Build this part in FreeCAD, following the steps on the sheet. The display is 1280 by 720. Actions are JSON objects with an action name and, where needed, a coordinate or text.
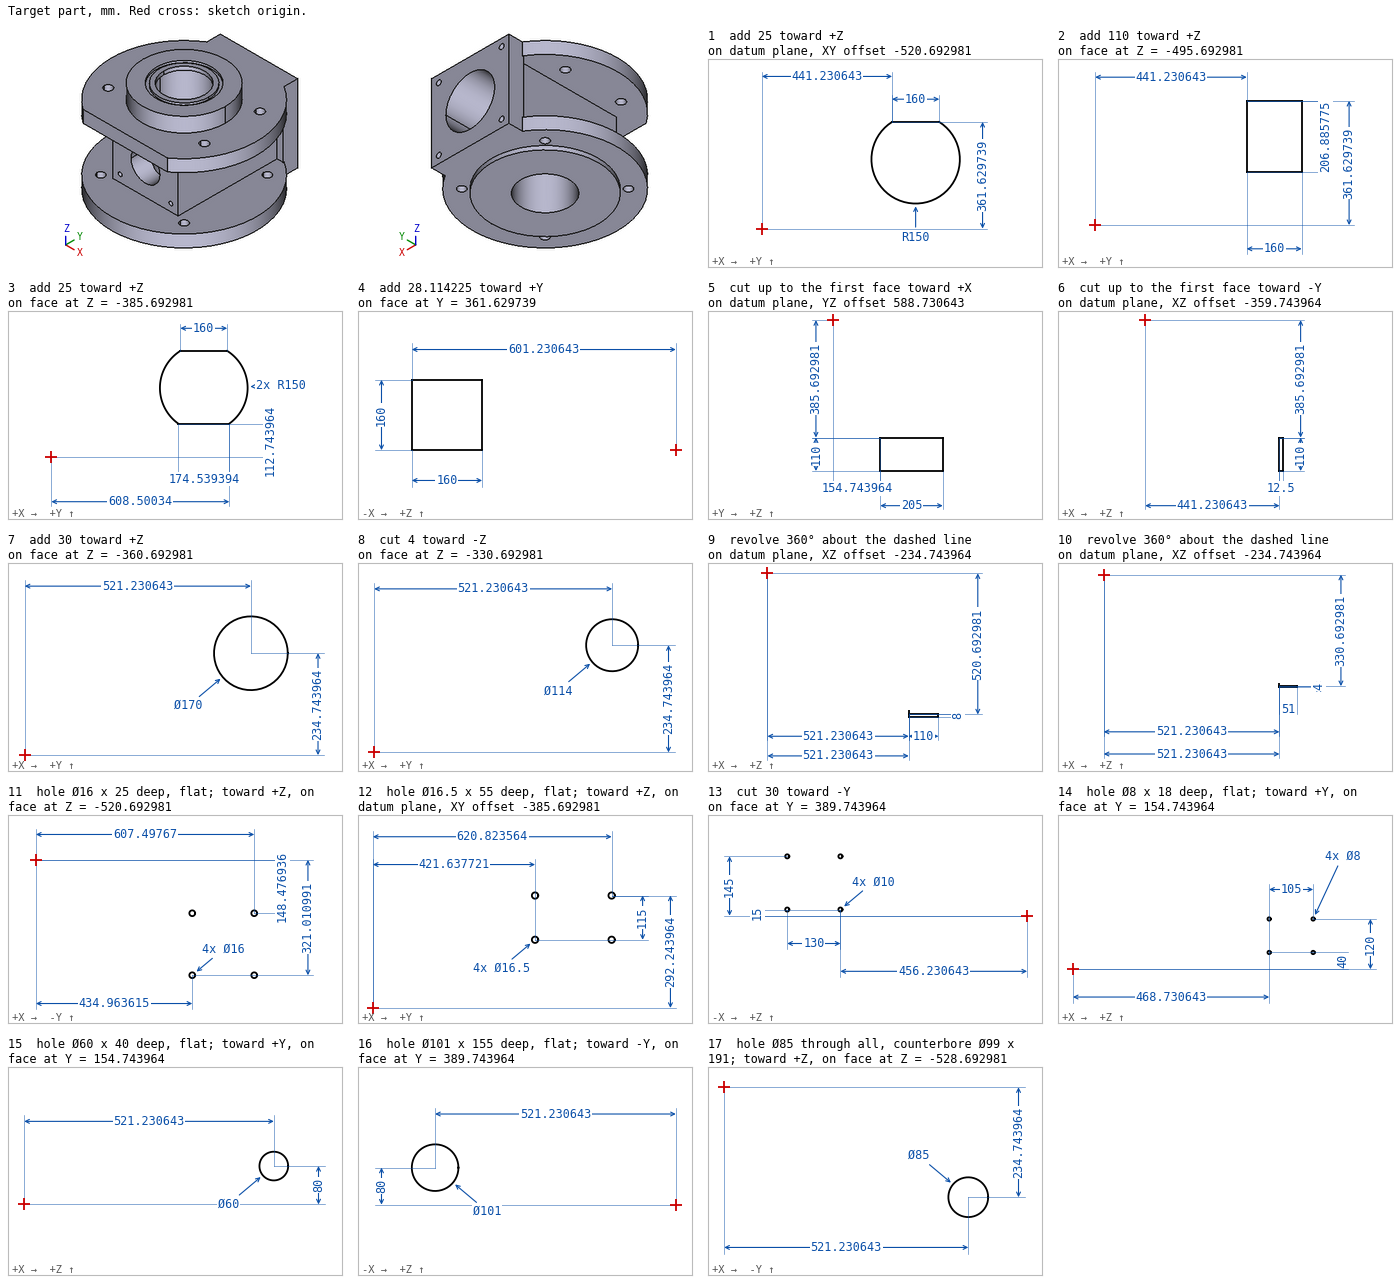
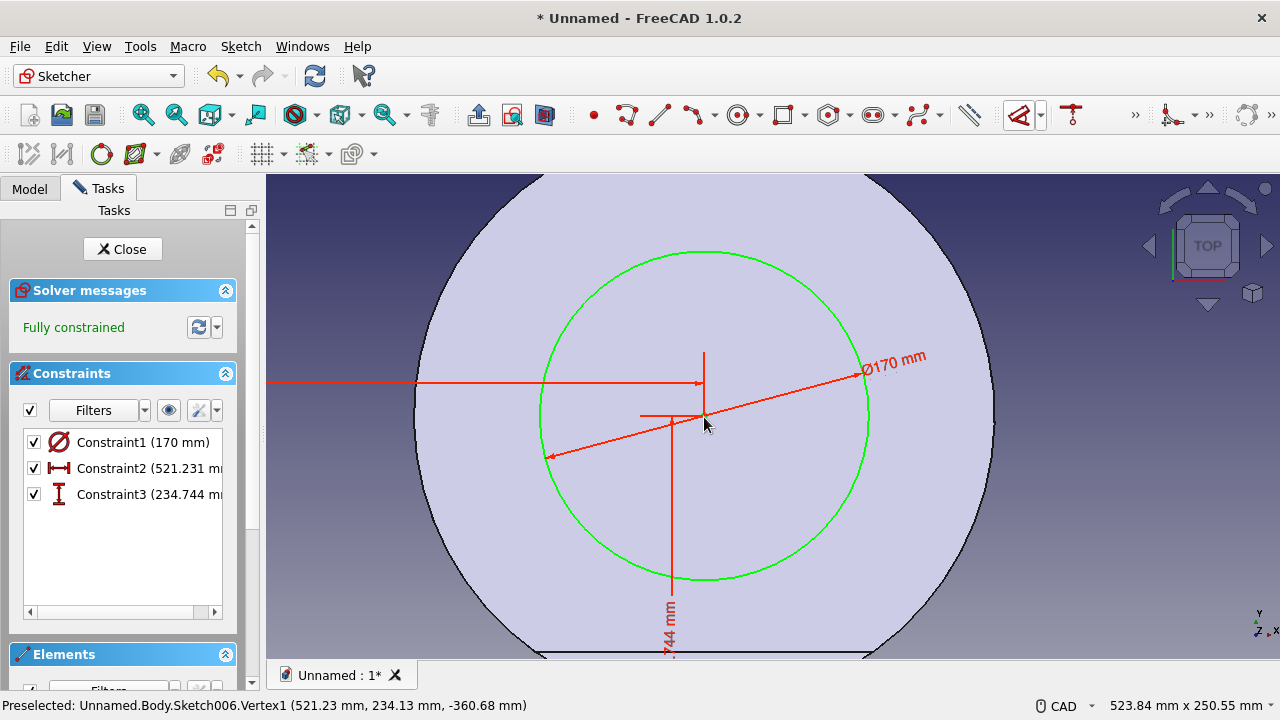
{"action": "left_click", "coordinate": [123, 249]}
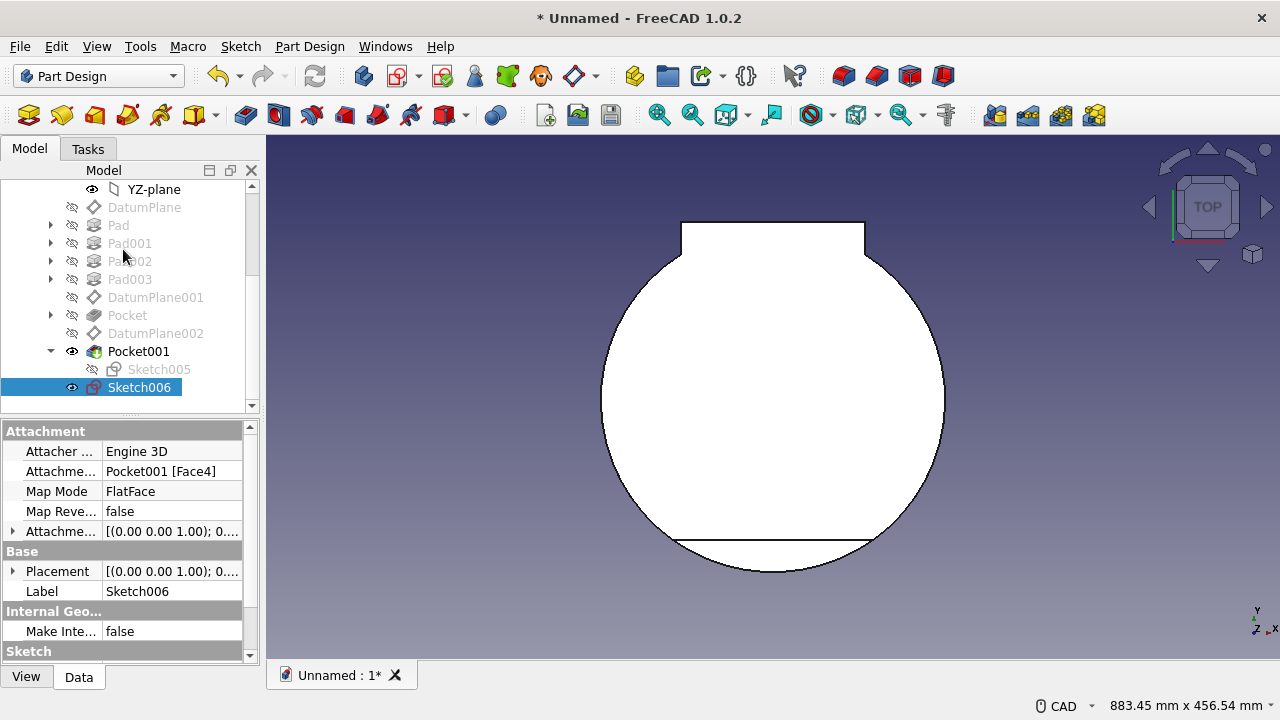
{"action": "left_click", "coordinate": [29, 116]}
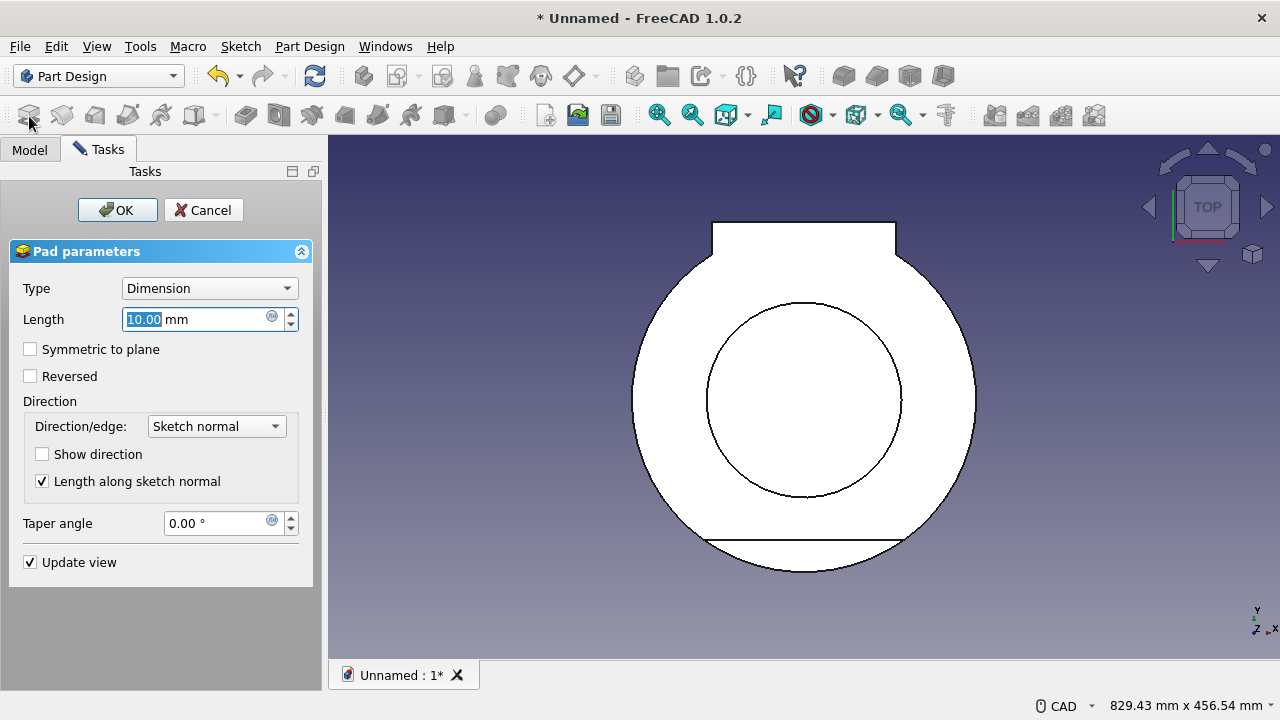
{"action": "type", "text": "30"}
{"action": "key", "text": "Tab"}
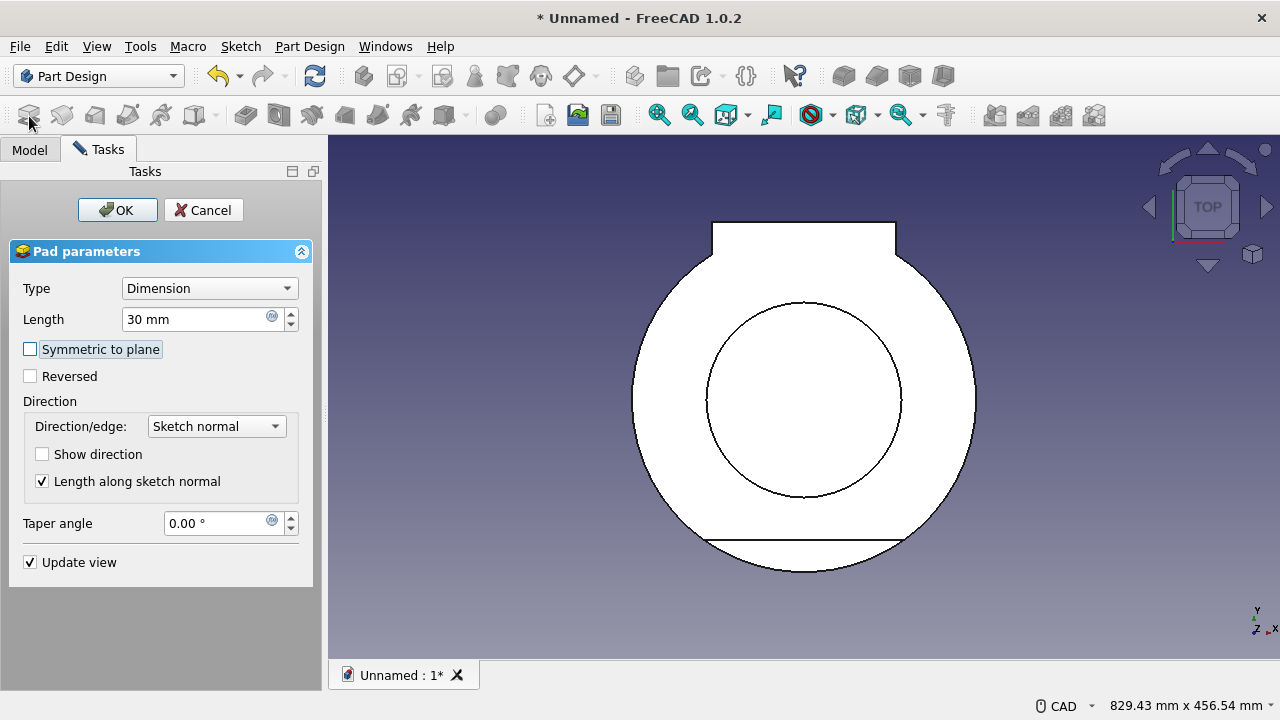
{"action": "left_click", "coordinate": [118, 210]}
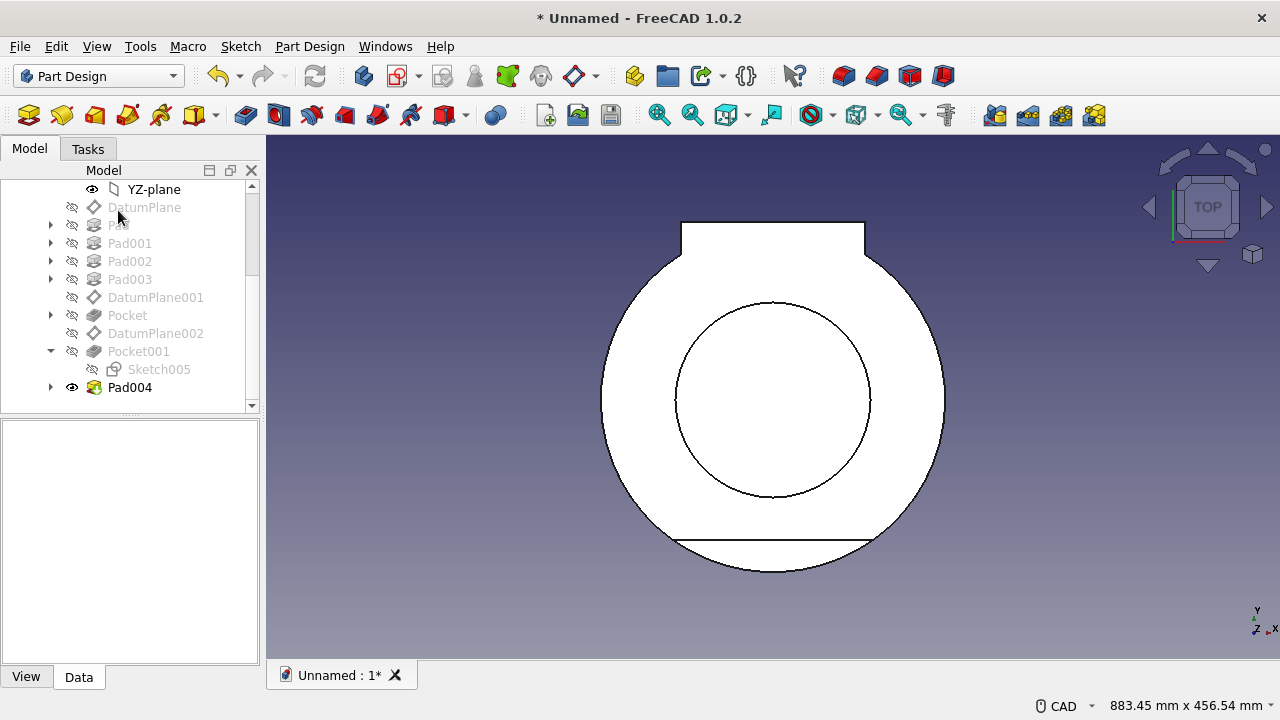
{"action": "left_click", "coordinate": [773, 399]}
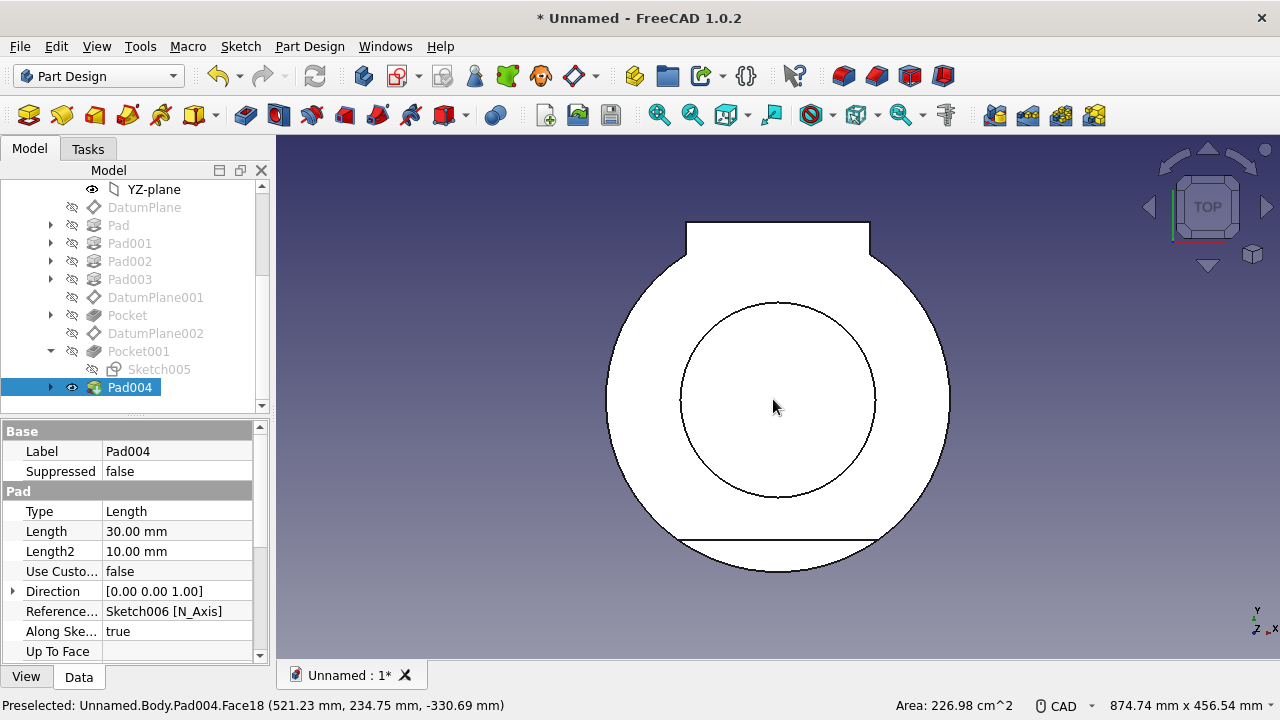
{"action": "left_click", "coordinate": [396, 76]}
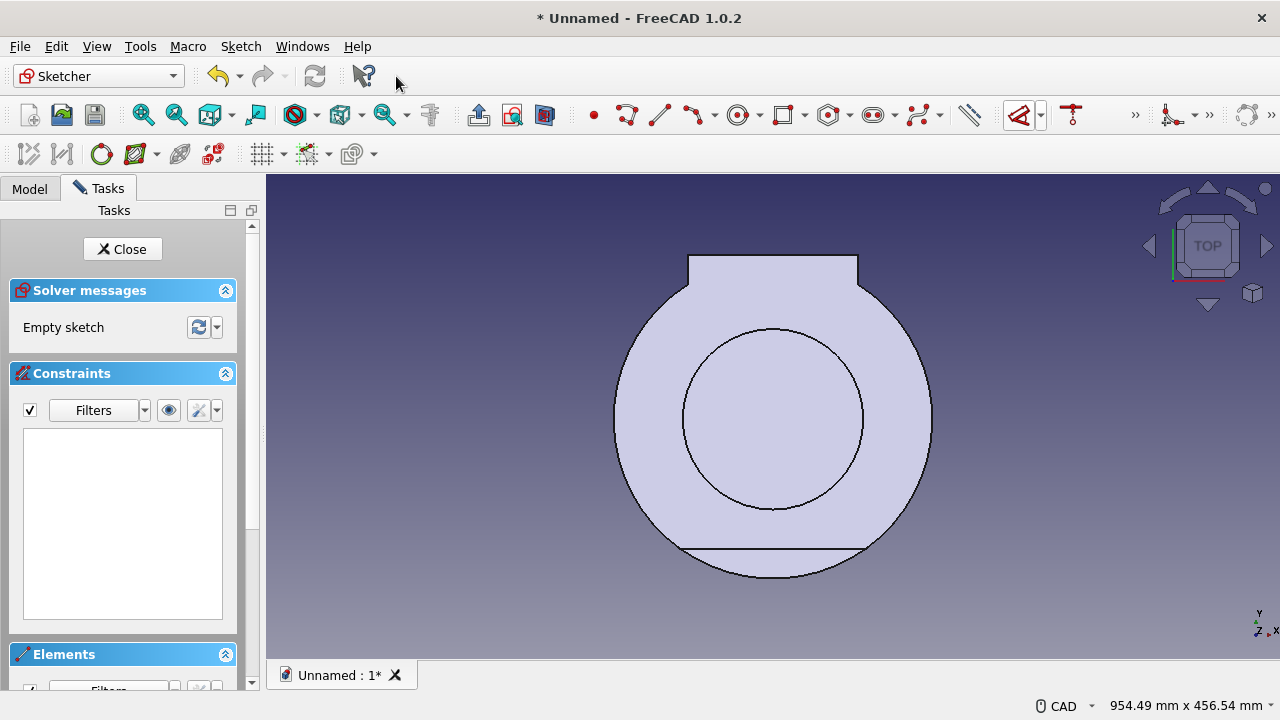
{"action": "scroll", "coordinate": [813, 421], "scroll_direction": "up", "scroll_amount": 5}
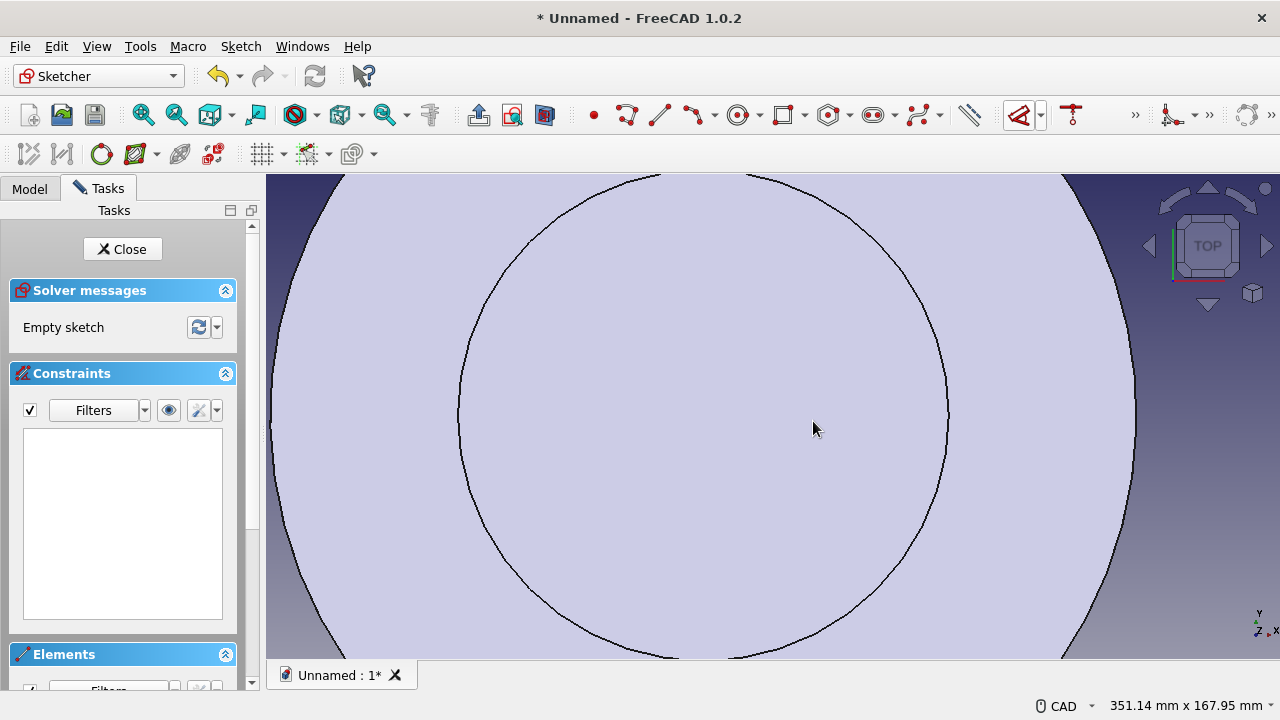
{"action": "left_click", "coordinate": [738, 116]}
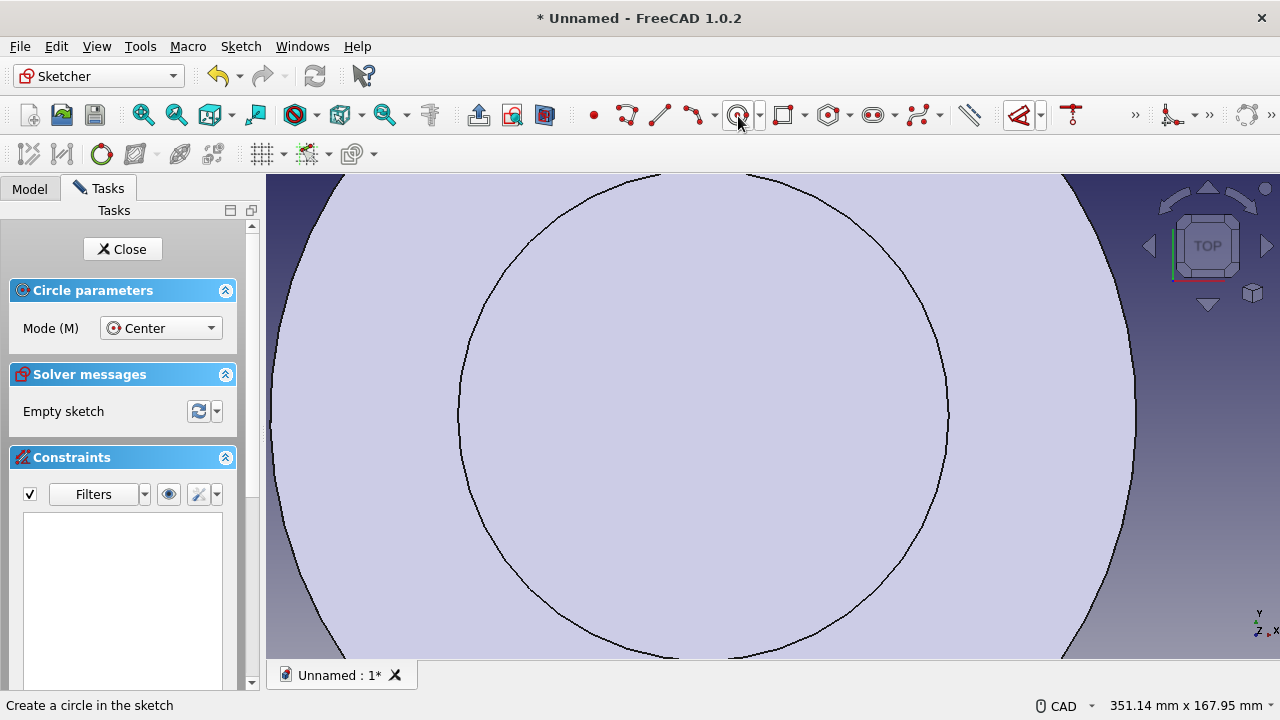
{"action": "left_click", "coordinate": [703, 415]}
{"action": "left_click", "coordinate": [820, 299]}
{"action": "key", "text": "Escape"}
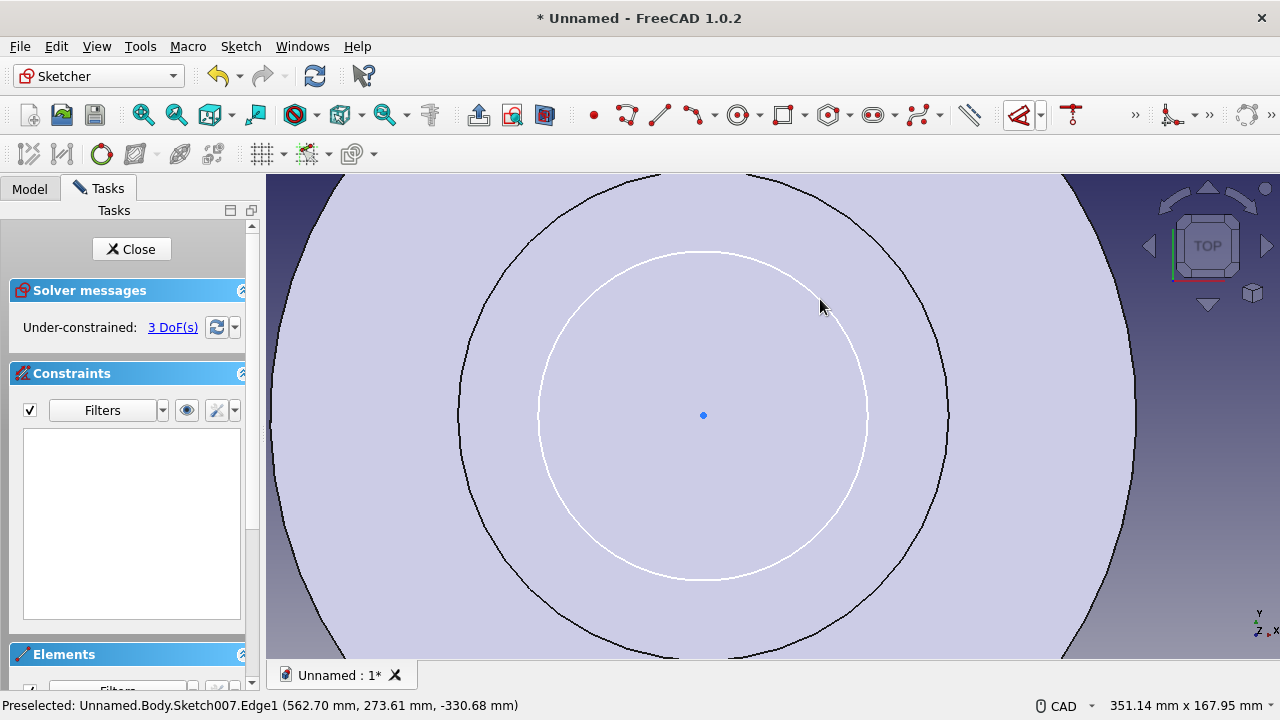
{"action": "left_click", "coordinate": [819, 299]}